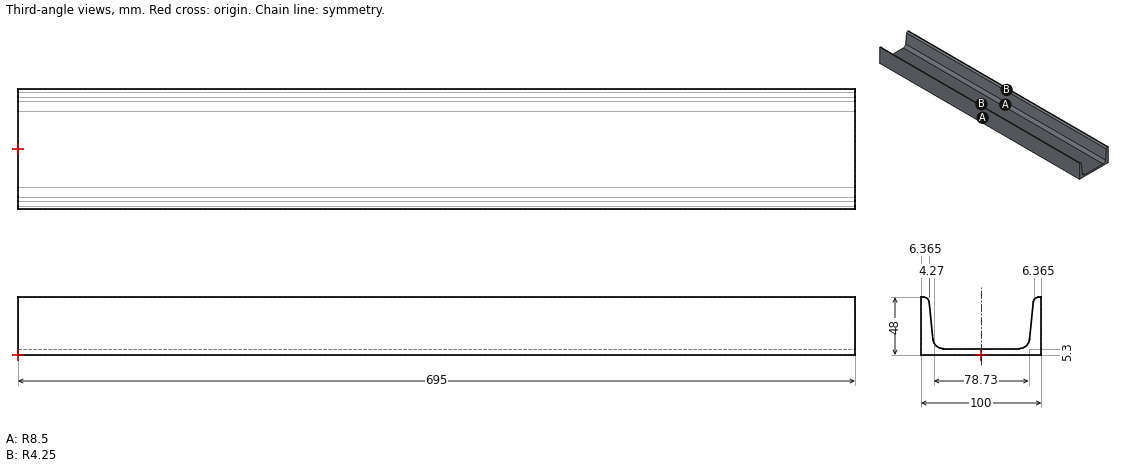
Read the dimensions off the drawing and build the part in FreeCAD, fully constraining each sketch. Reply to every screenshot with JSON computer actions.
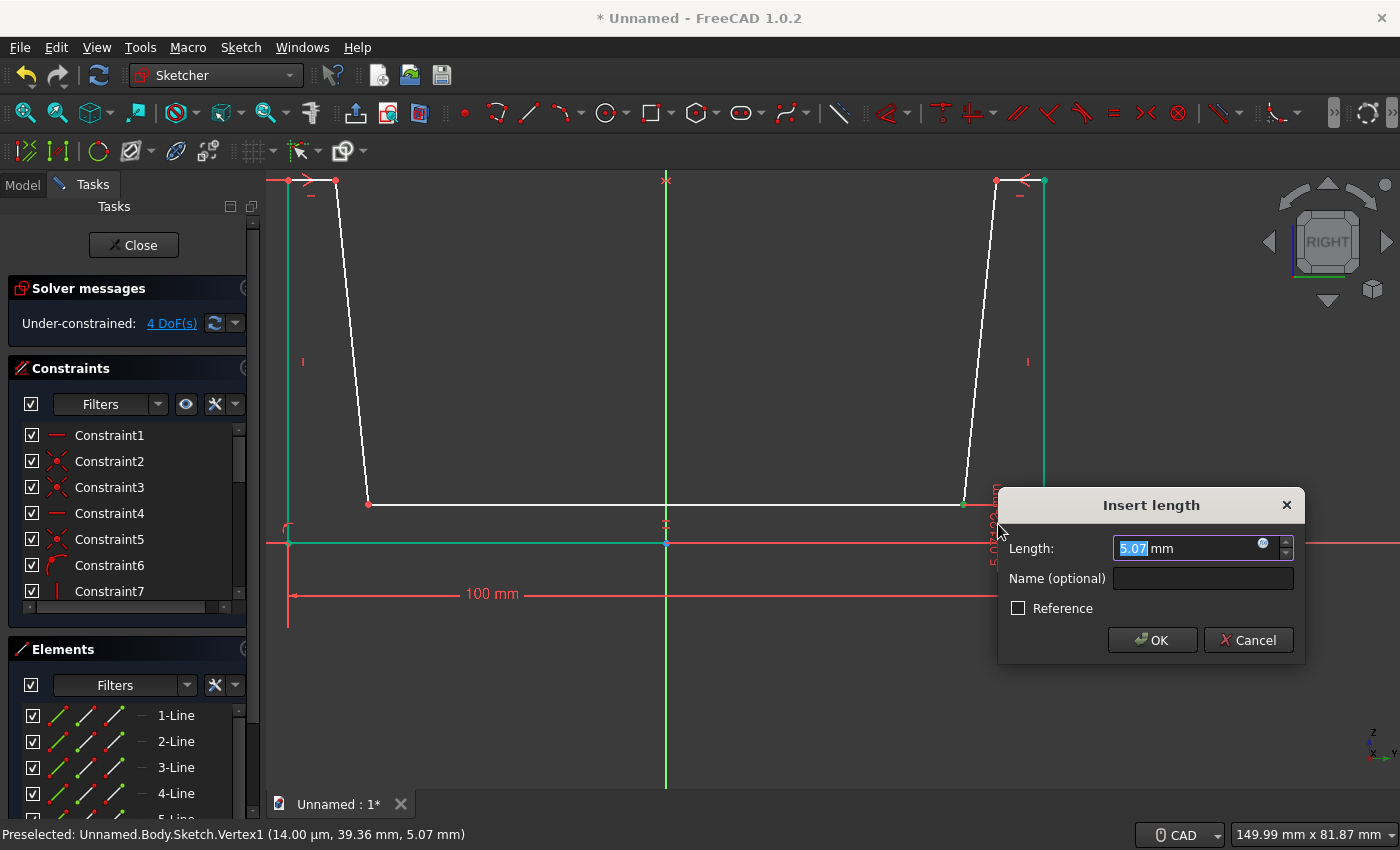
{"action": "type", "text": "5.3"}
{"action": "key", "text": "Return"}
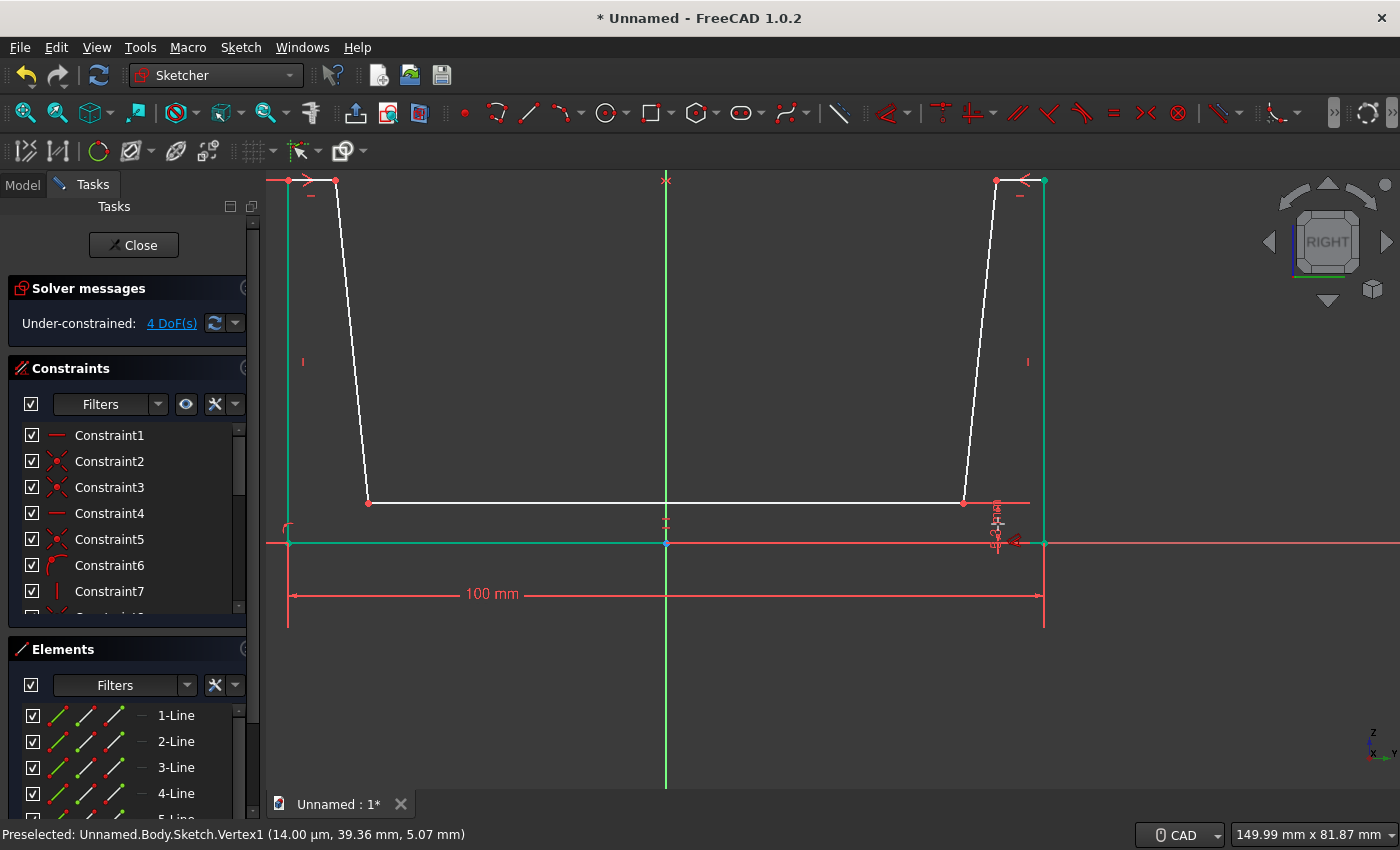
{"action": "left_click", "coordinate": [785, 503]}
{"action": "left_click", "coordinate": [529, 469]}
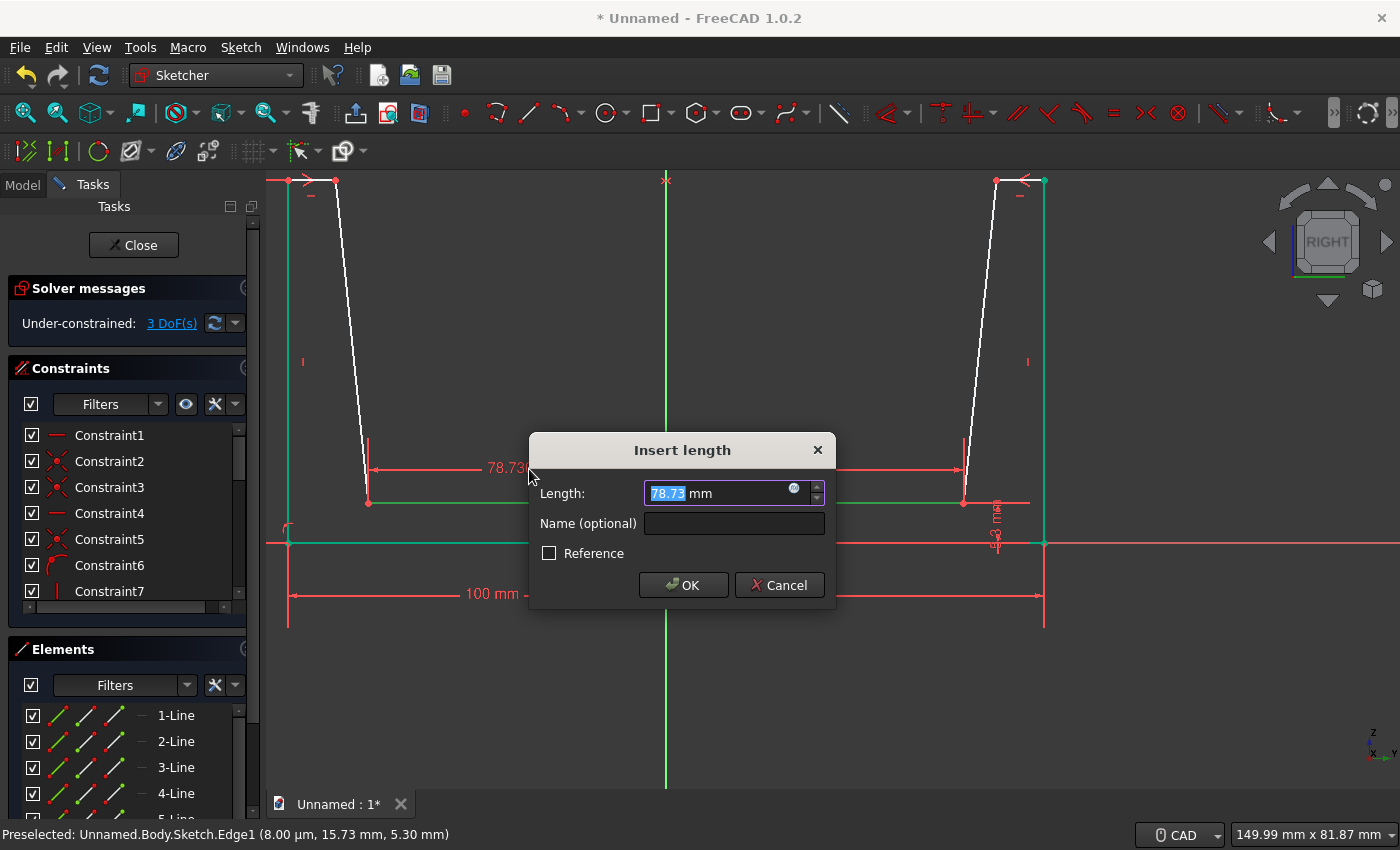
{"action": "type", "text": "78.73"}
{"action": "key", "text": "Return"}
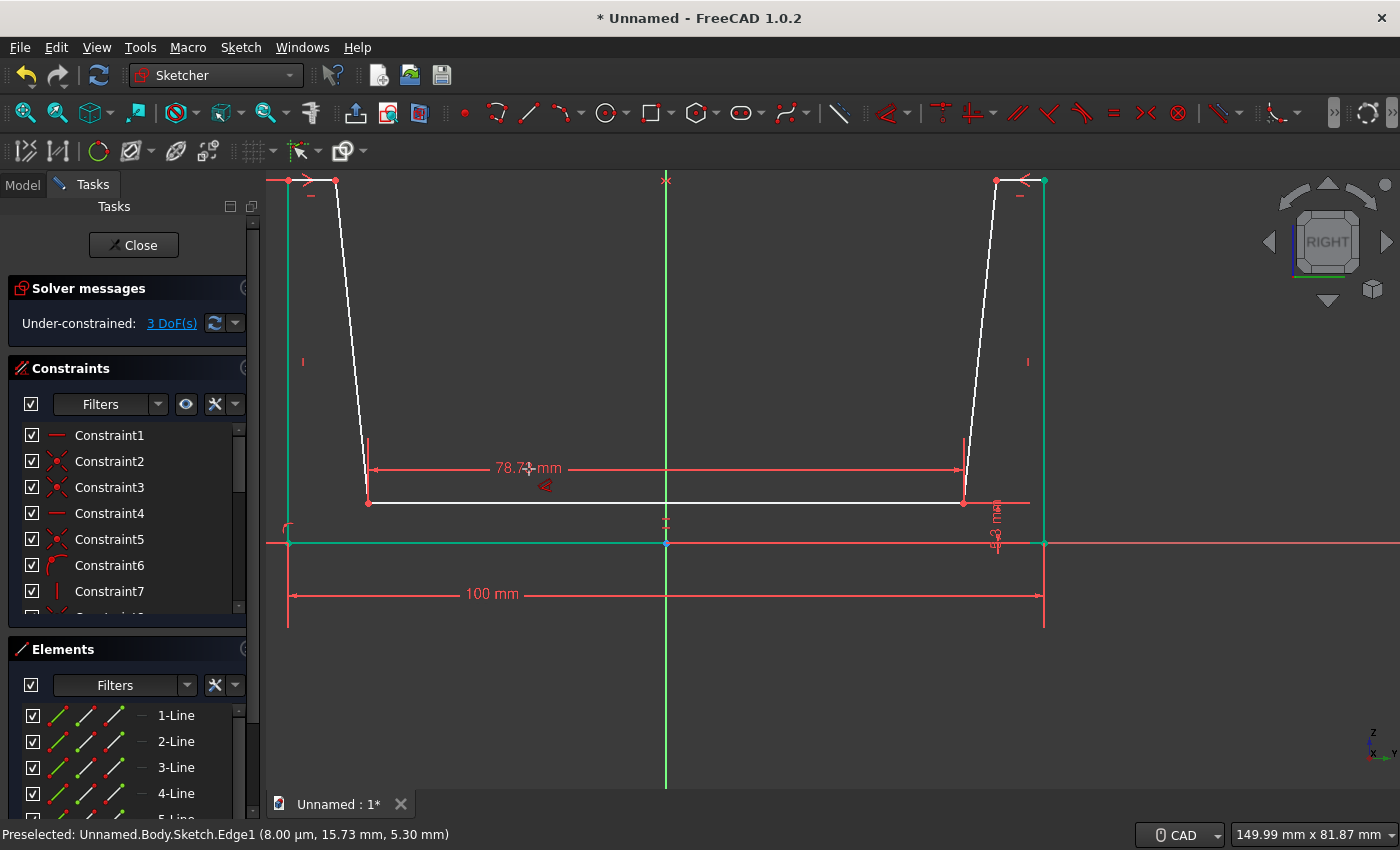
{"action": "scroll", "coordinate": [1209, 761], "scroll_direction": "down", "scroll_amount": 1}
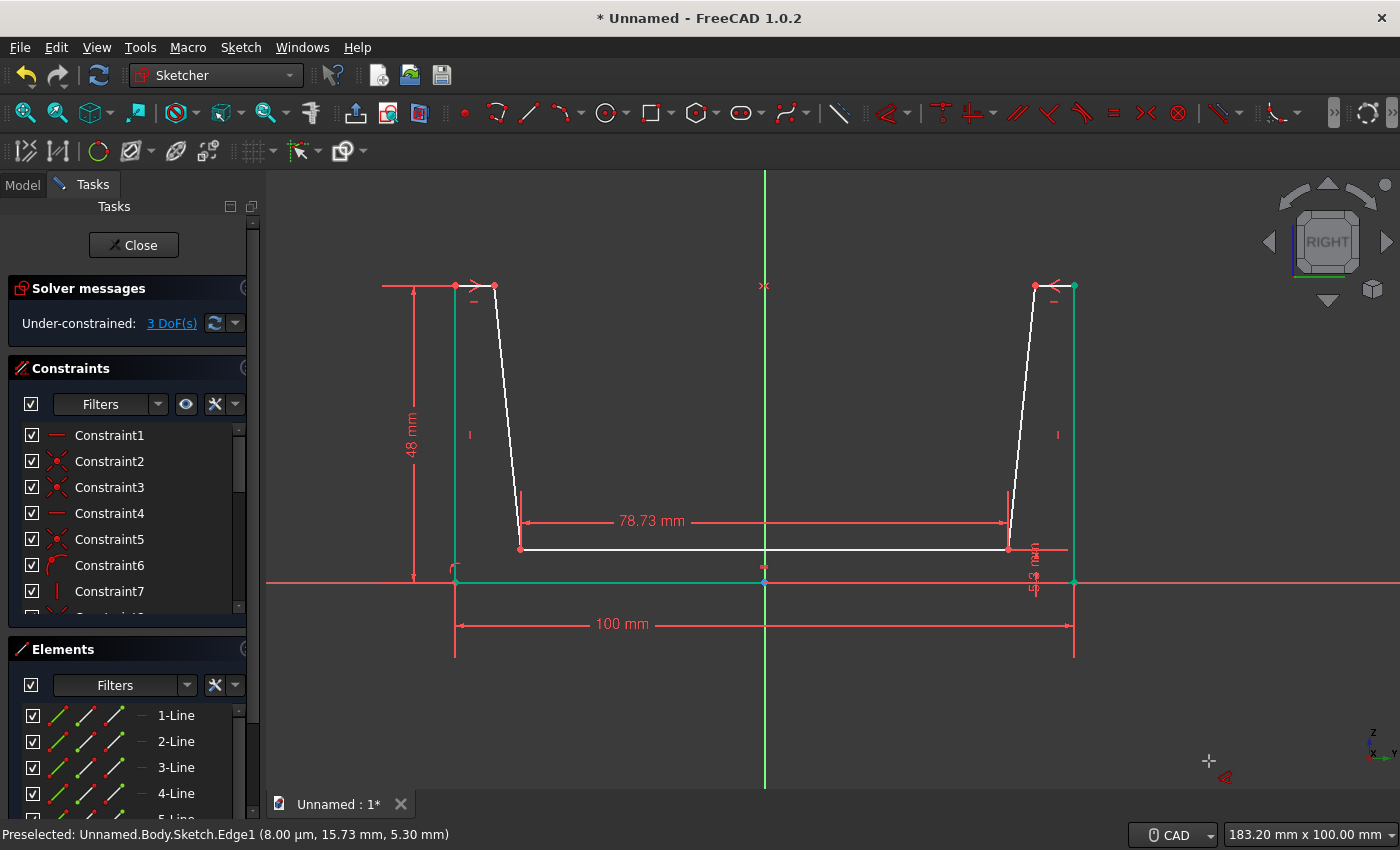
{"action": "left_click", "coordinate": [482, 286]}
{"action": "left_click", "coordinate": [475, 252]}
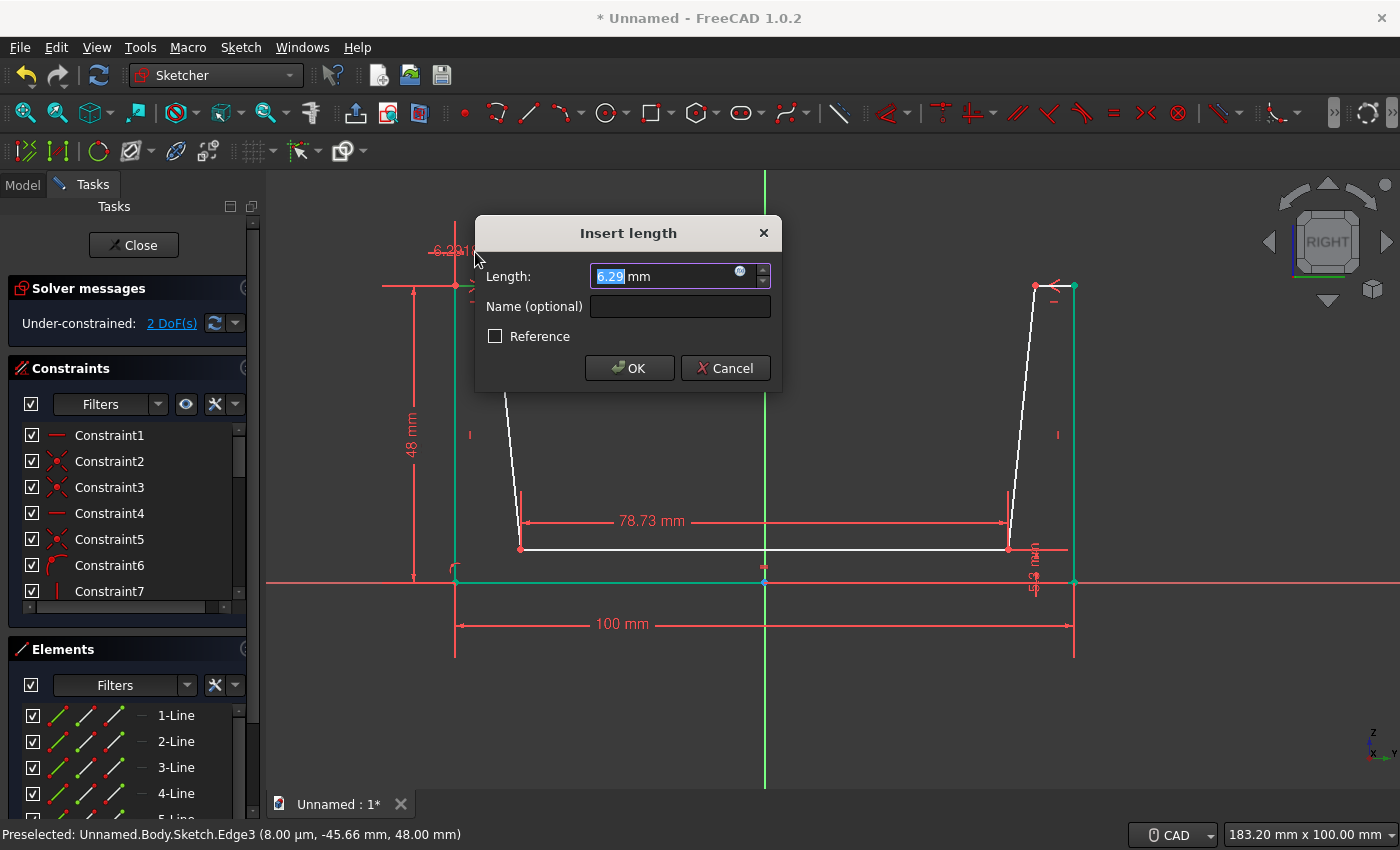
{"action": "type", "text": "6.365"}
{"action": "key", "text": "Return"}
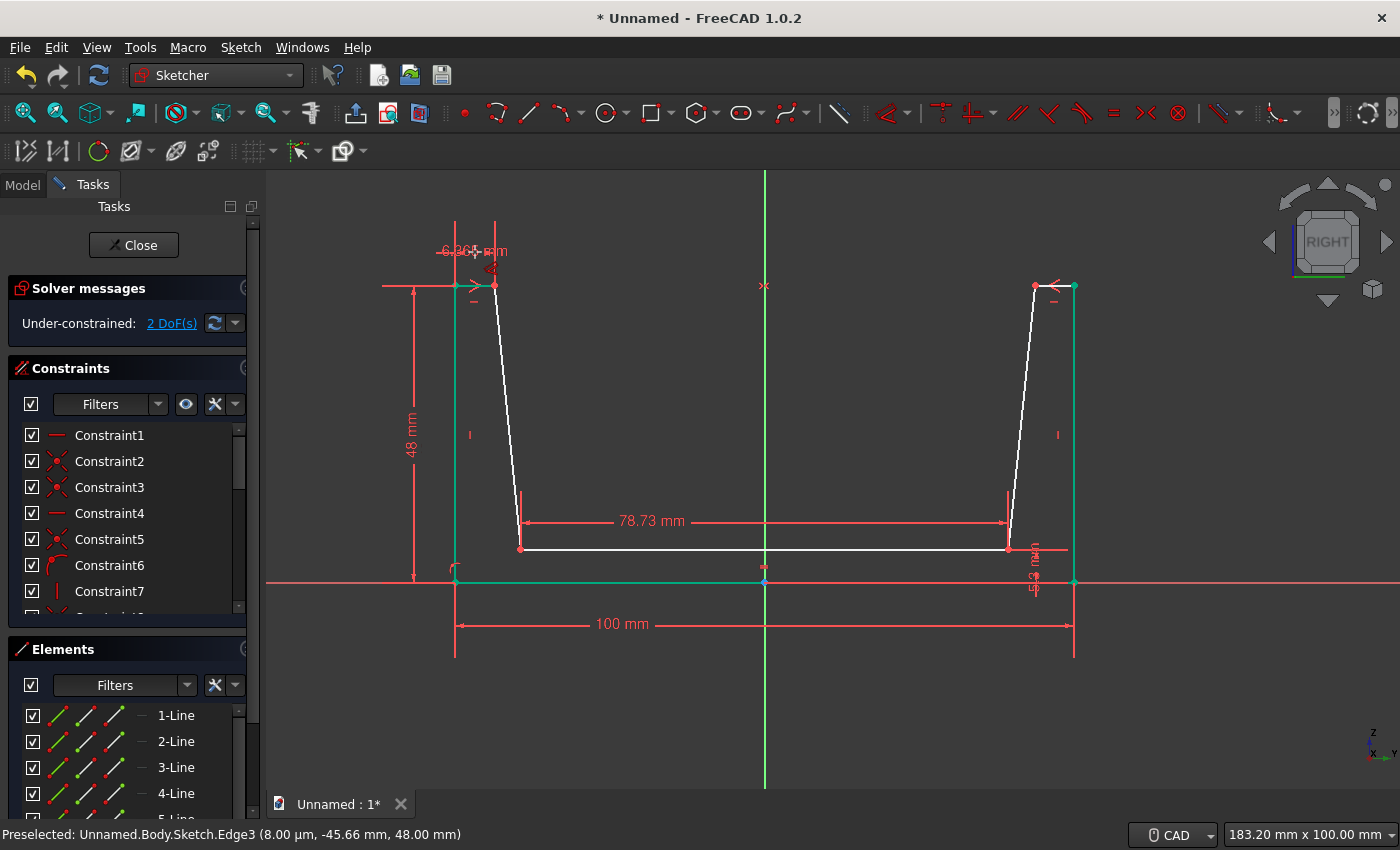
{"action": "left_click", "coordinate": [1062, 286]}
{"action": "left_click", "coordinate": [1055, 252]}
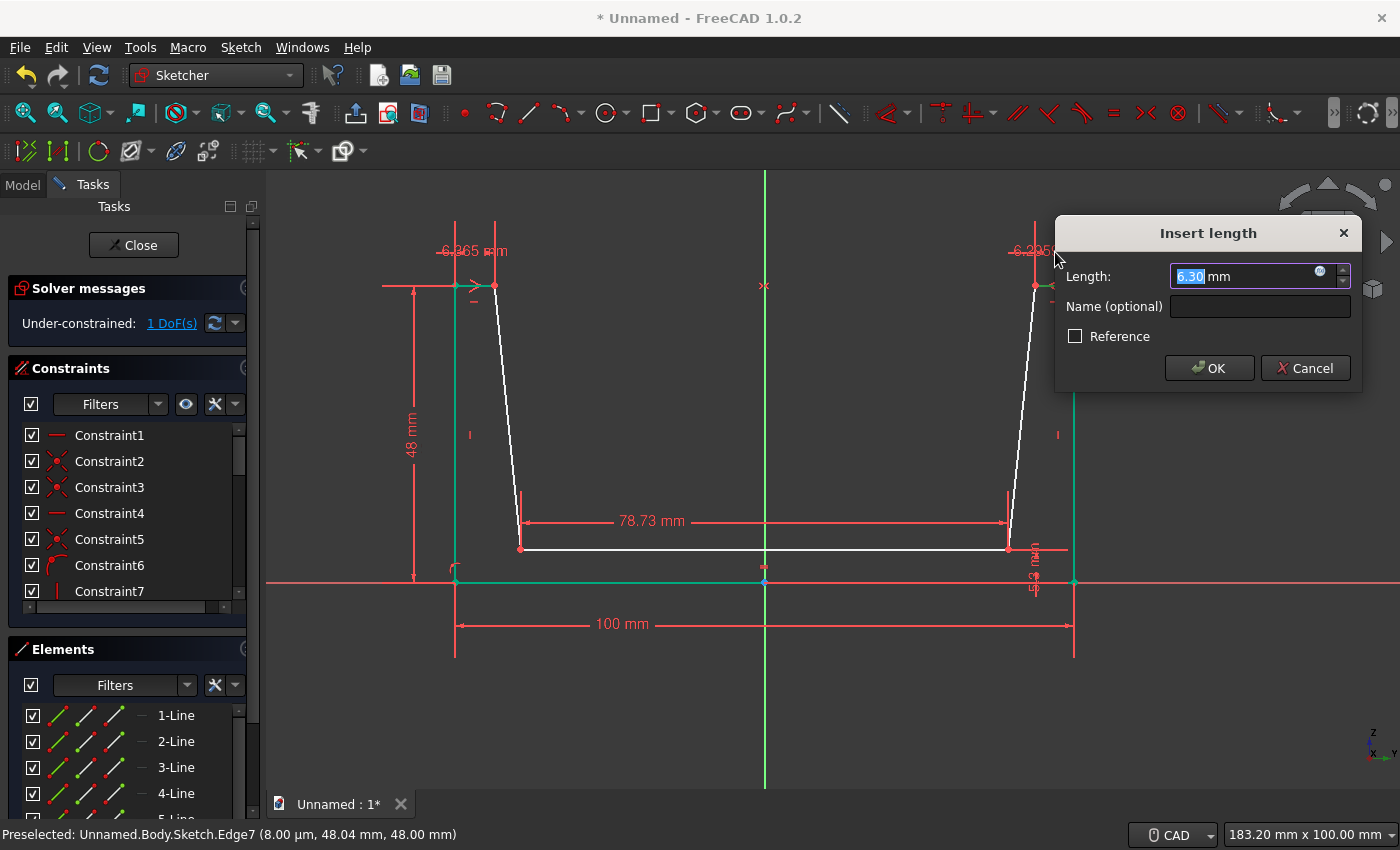
{"action": "type", "text": "6.365"}
{"action": "key", "text": "Return"}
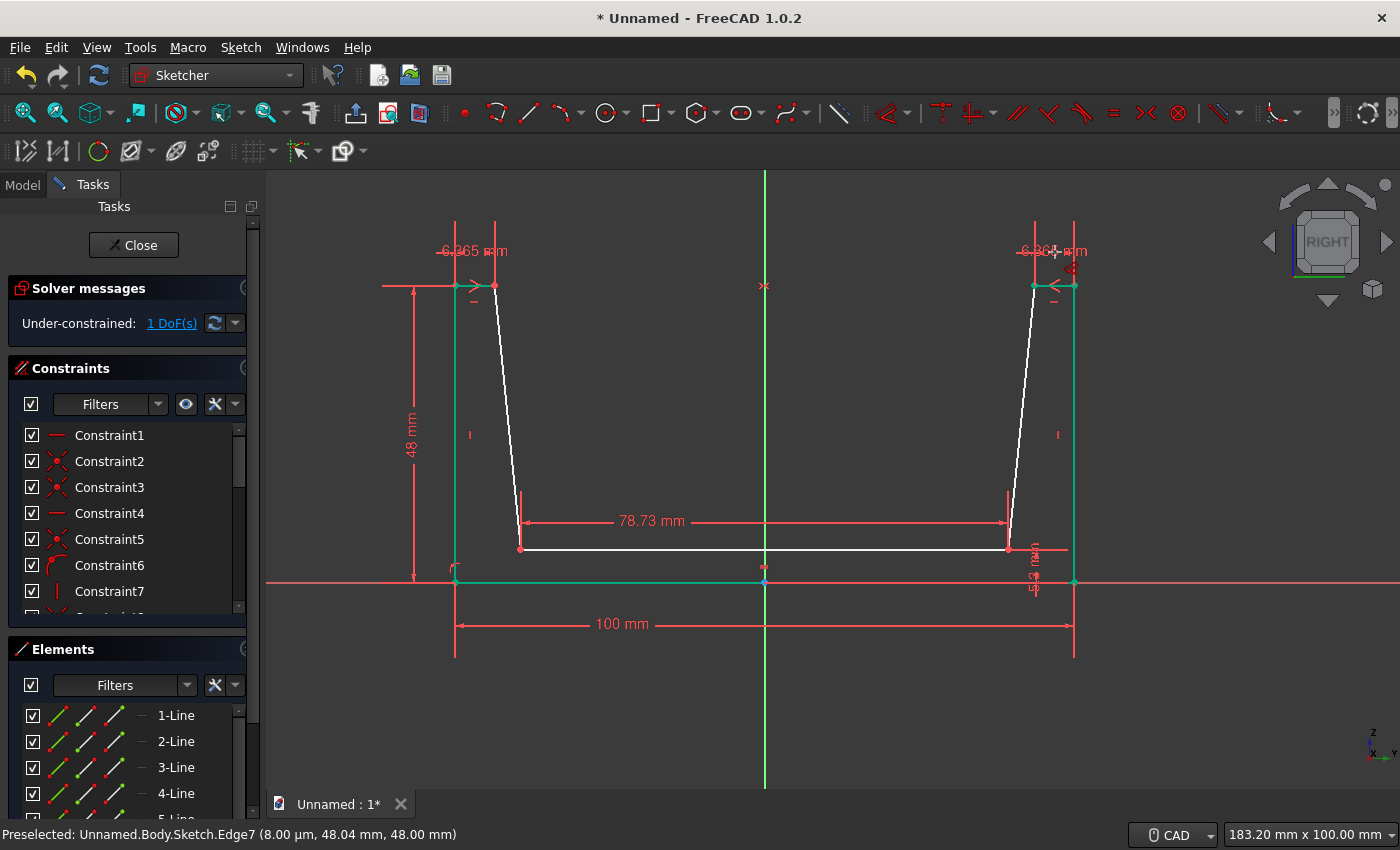
{"action": "scroll", "coordinate": [513, 471], "scroll_direction": "up", "scroll_amount": 3}